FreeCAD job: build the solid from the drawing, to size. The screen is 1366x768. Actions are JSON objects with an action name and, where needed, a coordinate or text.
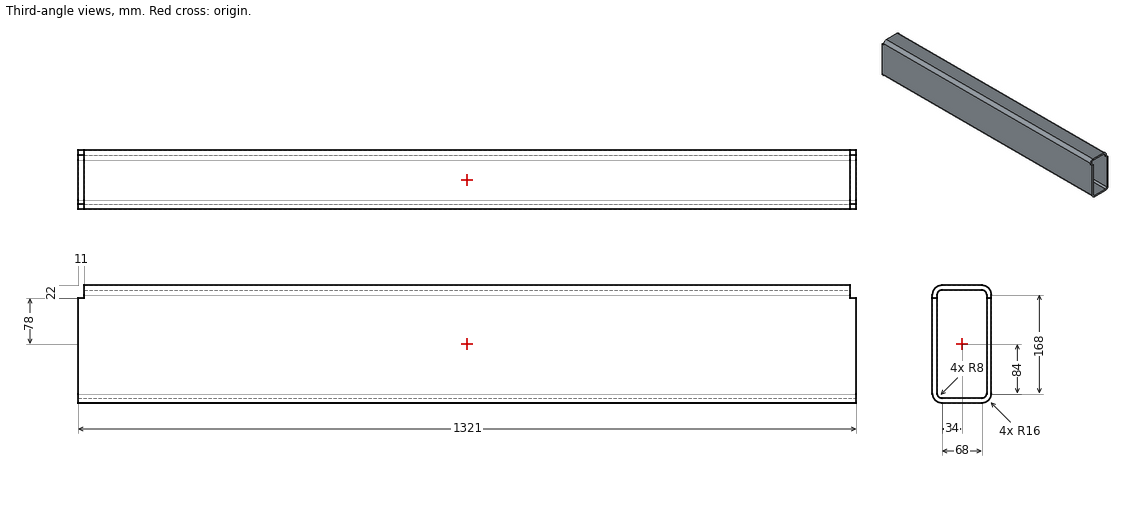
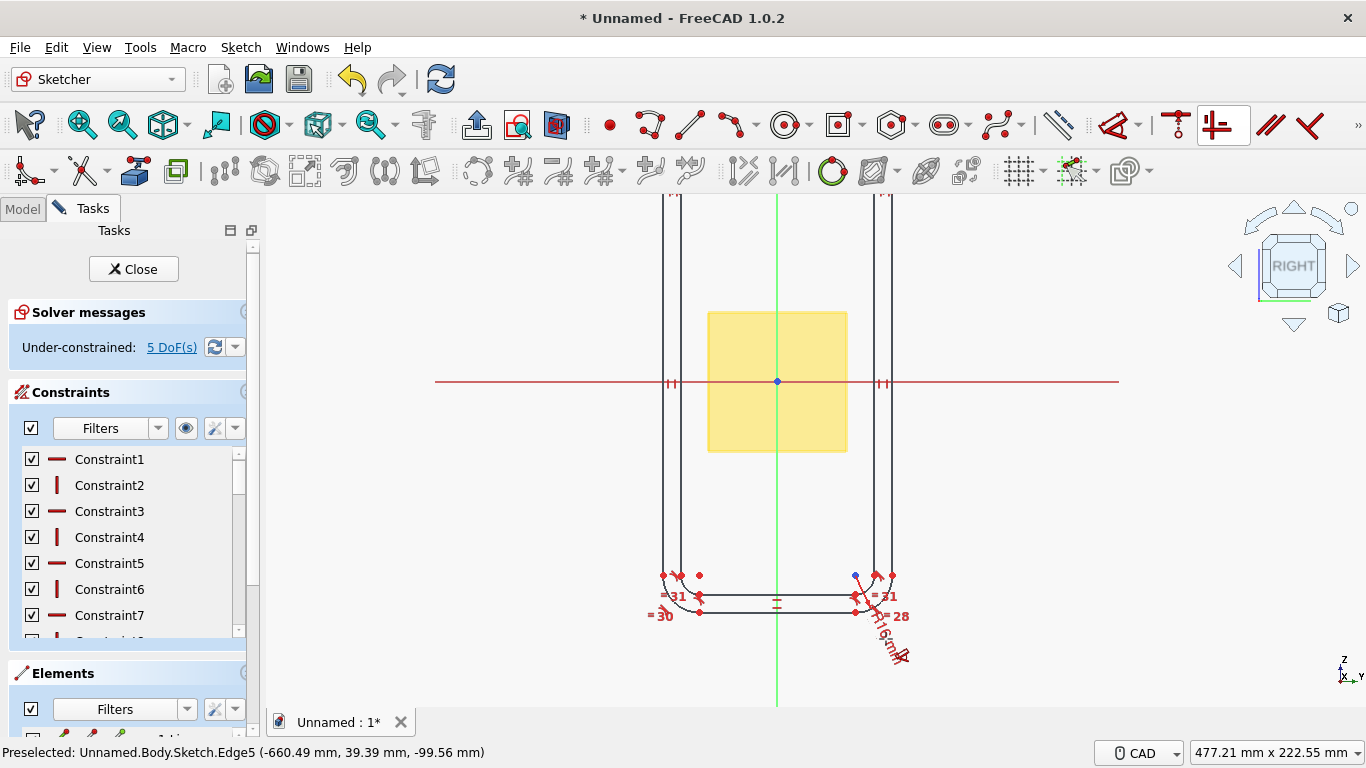
{"action": "scroll", "coordinate": [687, 589], "scroll_direction": "up", "scroll_amount": 4}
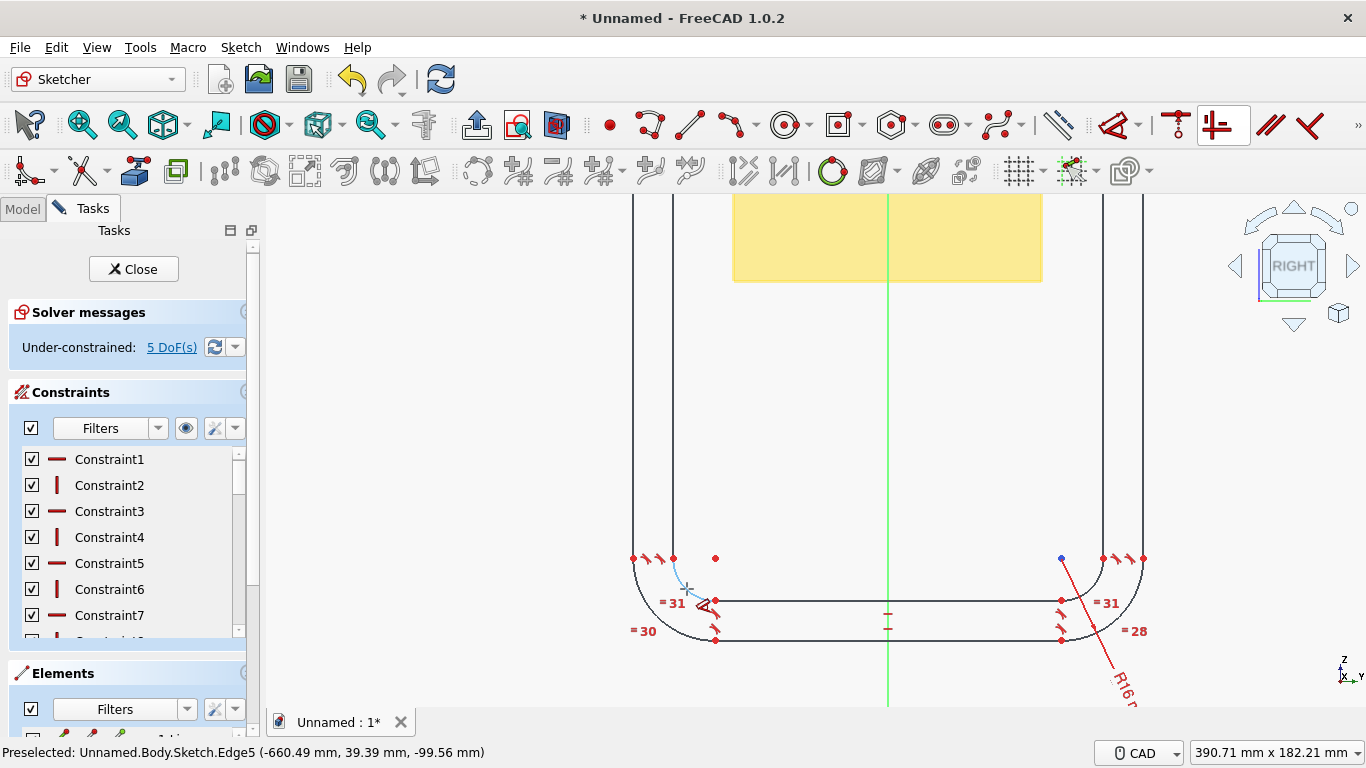
{"action": "left_click", "coordinate": [686, 589]}
{"action": "left_click", "coordinate": [767, 506]}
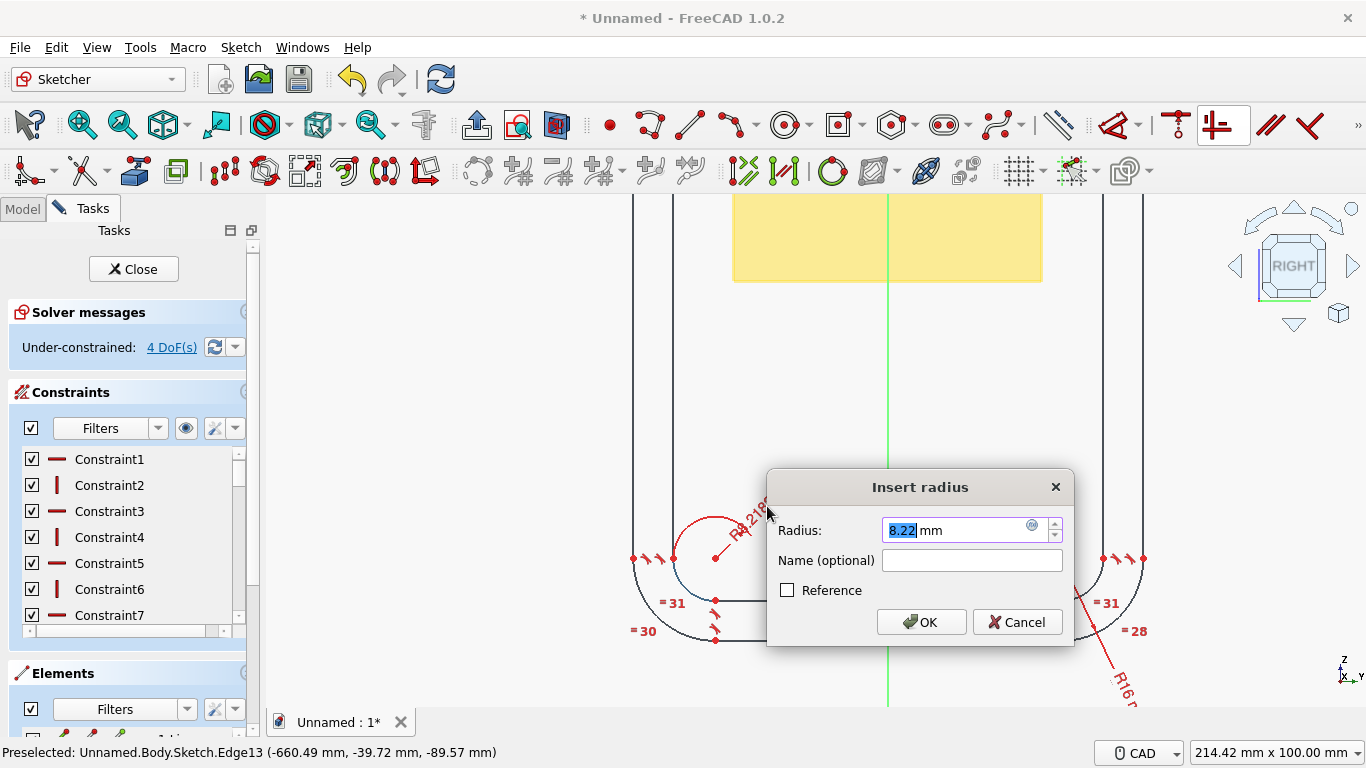
{"action": "type", "text": "8"}
{"action": "key", "text": "Return"}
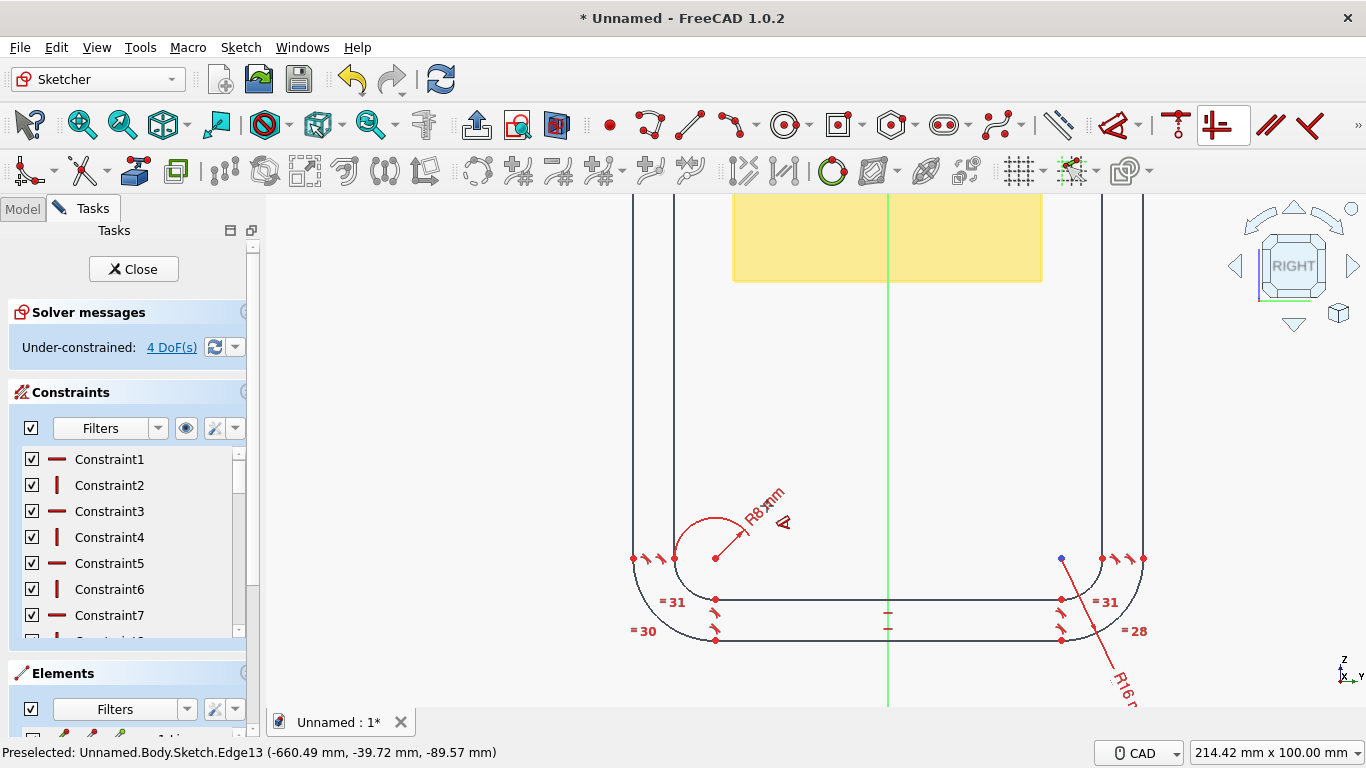
{"action": "left_click", "coordinate": [819, 641]}
{"action": "left_click", "coordinate": [809, 675]}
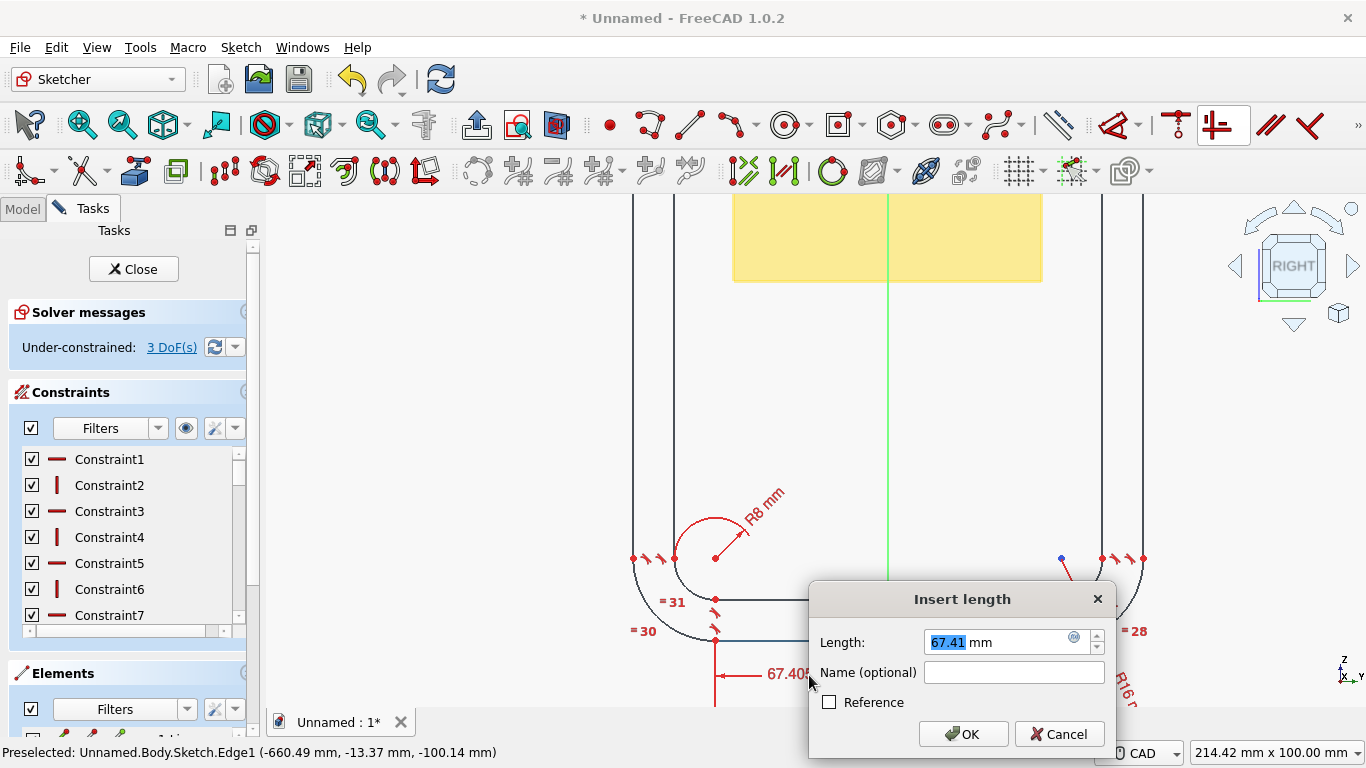
{"action": "type", "text": "68"}
{"action": "key", "text": "Return"}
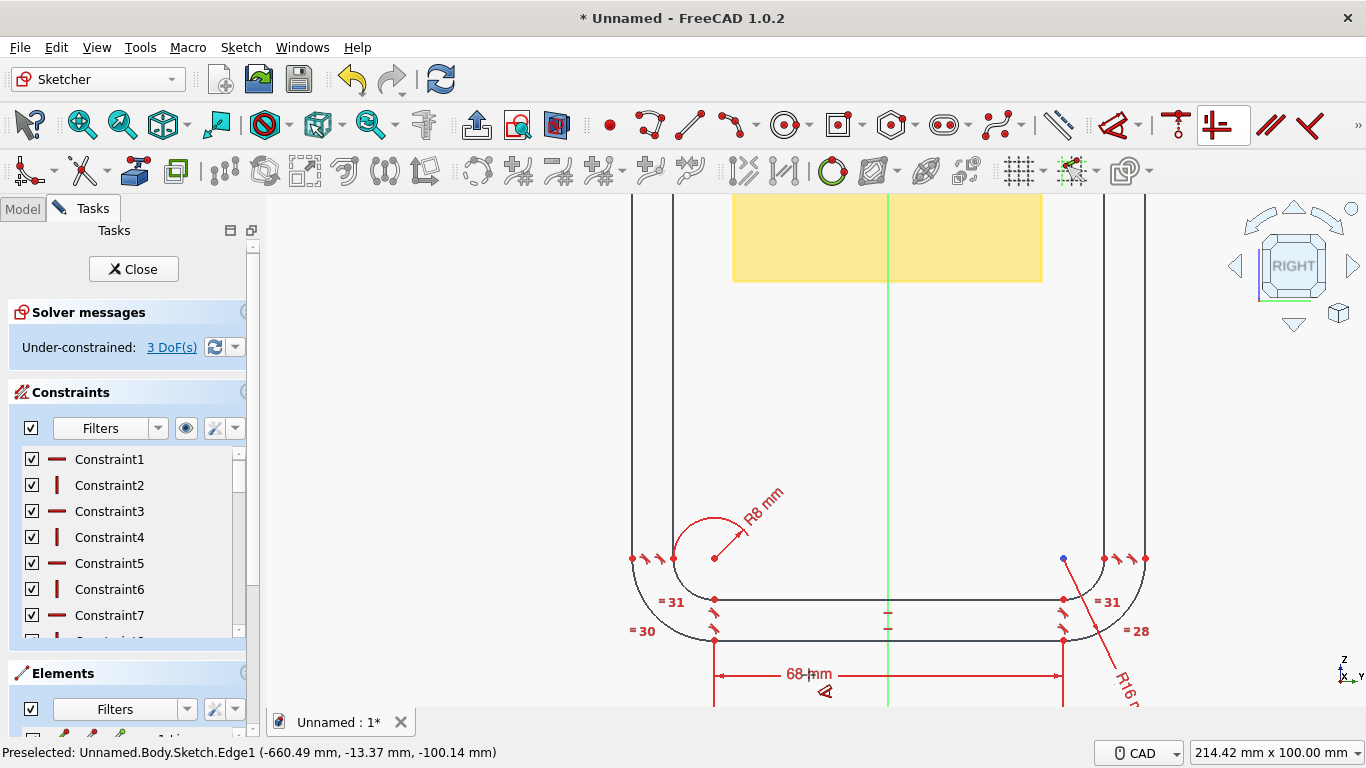
{"action": "left_click", "coordinate": [1145, 301]}
{"action": "left_click", "coordinate": [1179, 390]}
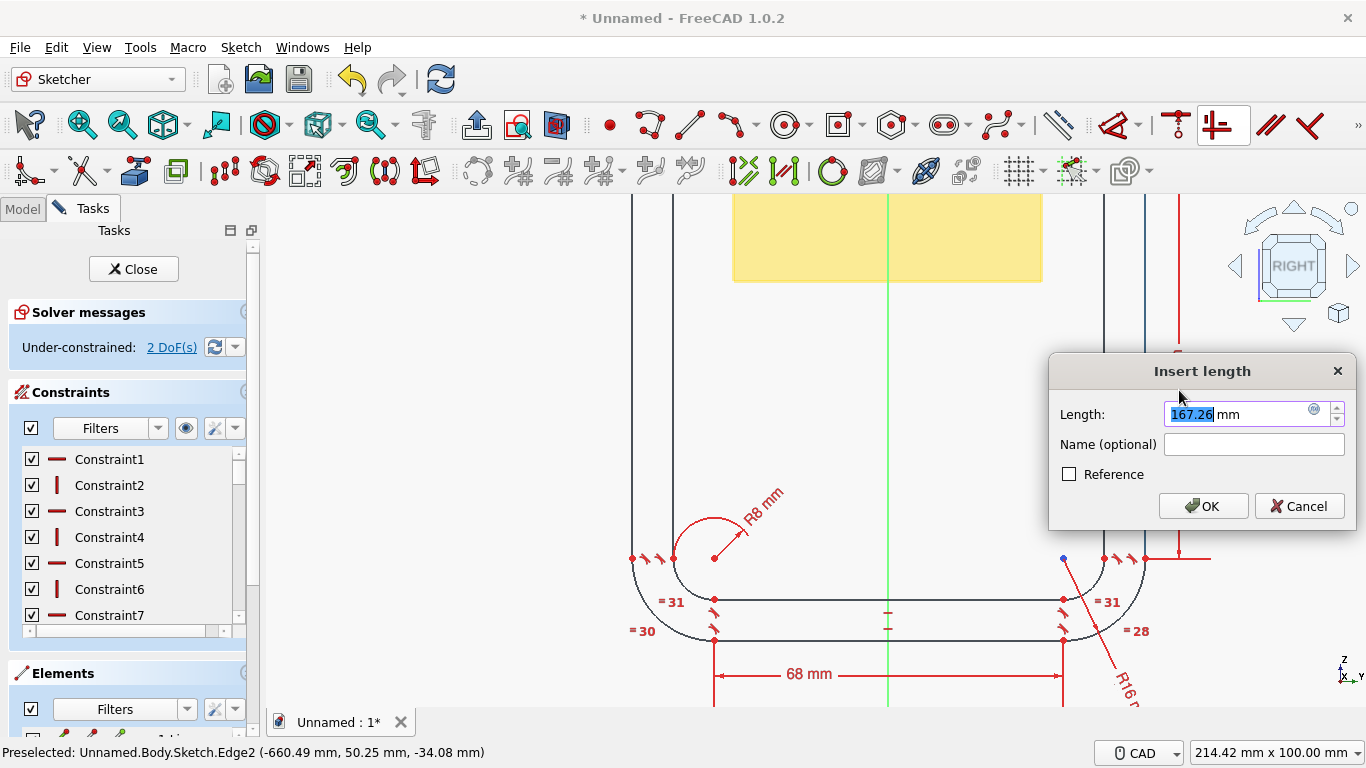
{"action": "type", "text": "168"}
{"action": "key", "text": "Return"}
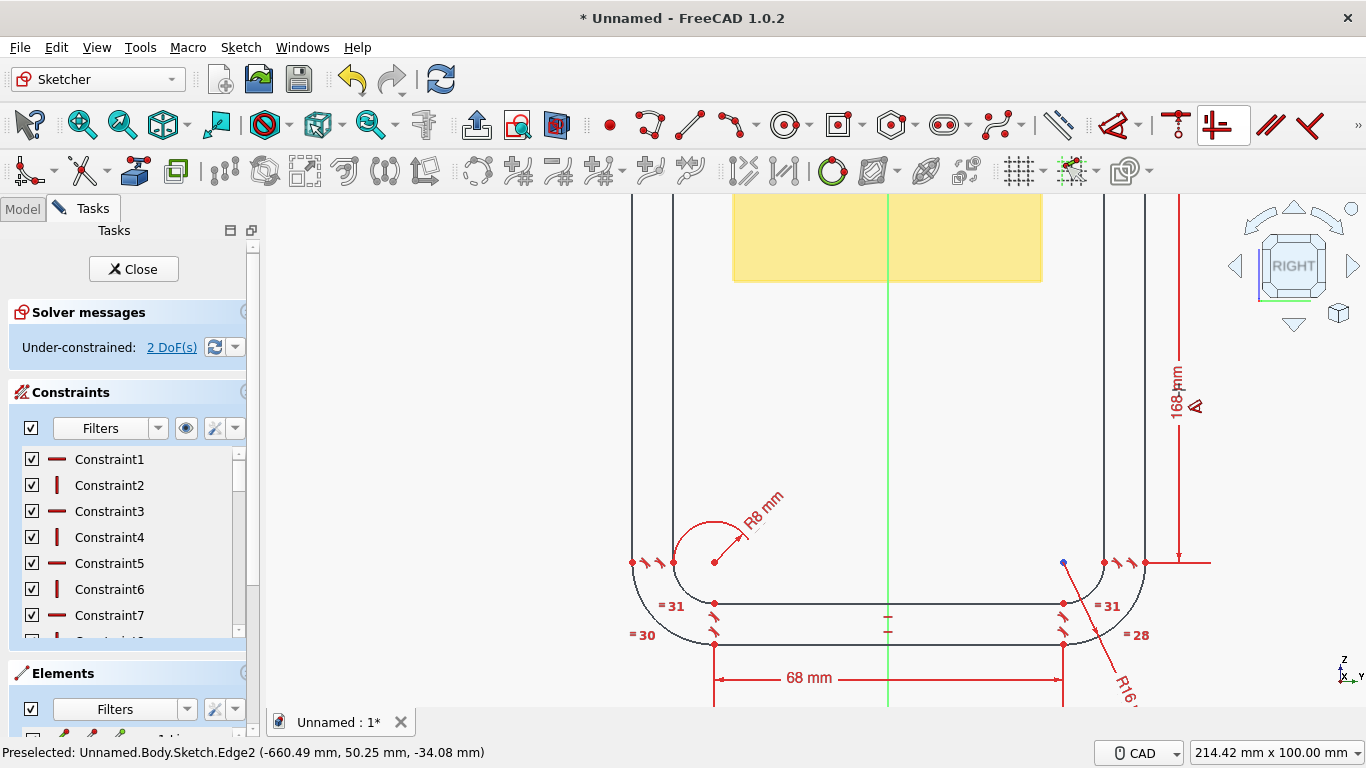
{"action": "left_click", "coordinate": [714, 645]}
{"action": "left_click", "coordinate": [761, 679]}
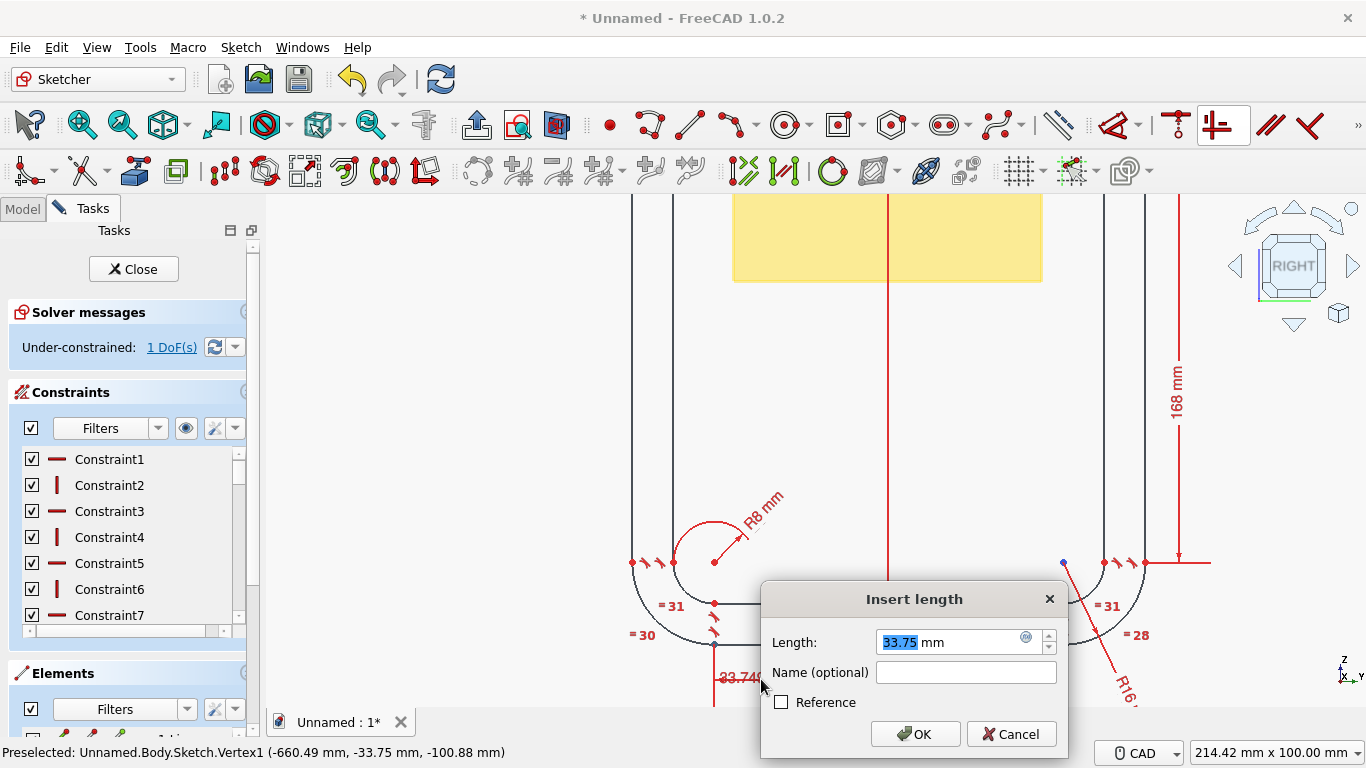
{"action": "type", "text": "34"}
{"action": "key", "text": "Return"}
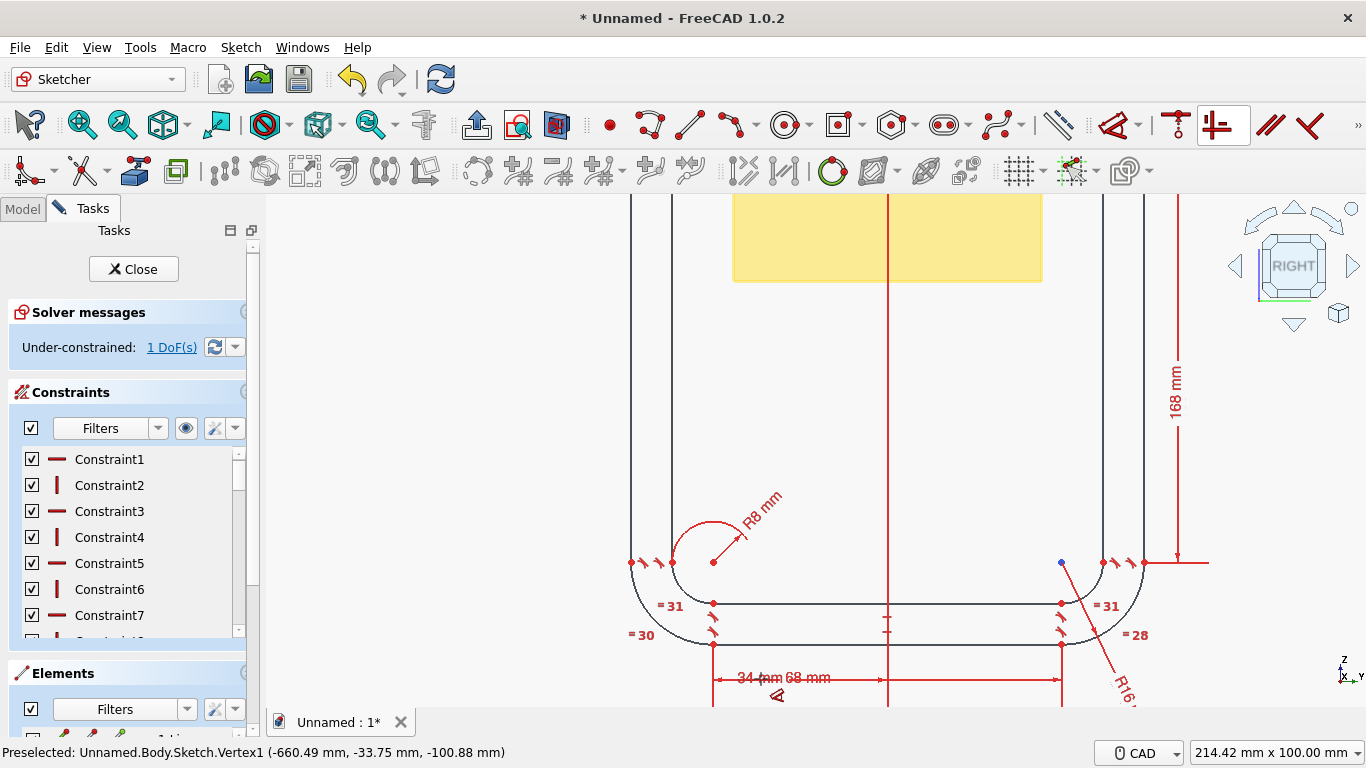
{"action": "left_click", "coordinate": [1144, 563]}
{"action": "left_click", "coordinate": [1178, 314]}